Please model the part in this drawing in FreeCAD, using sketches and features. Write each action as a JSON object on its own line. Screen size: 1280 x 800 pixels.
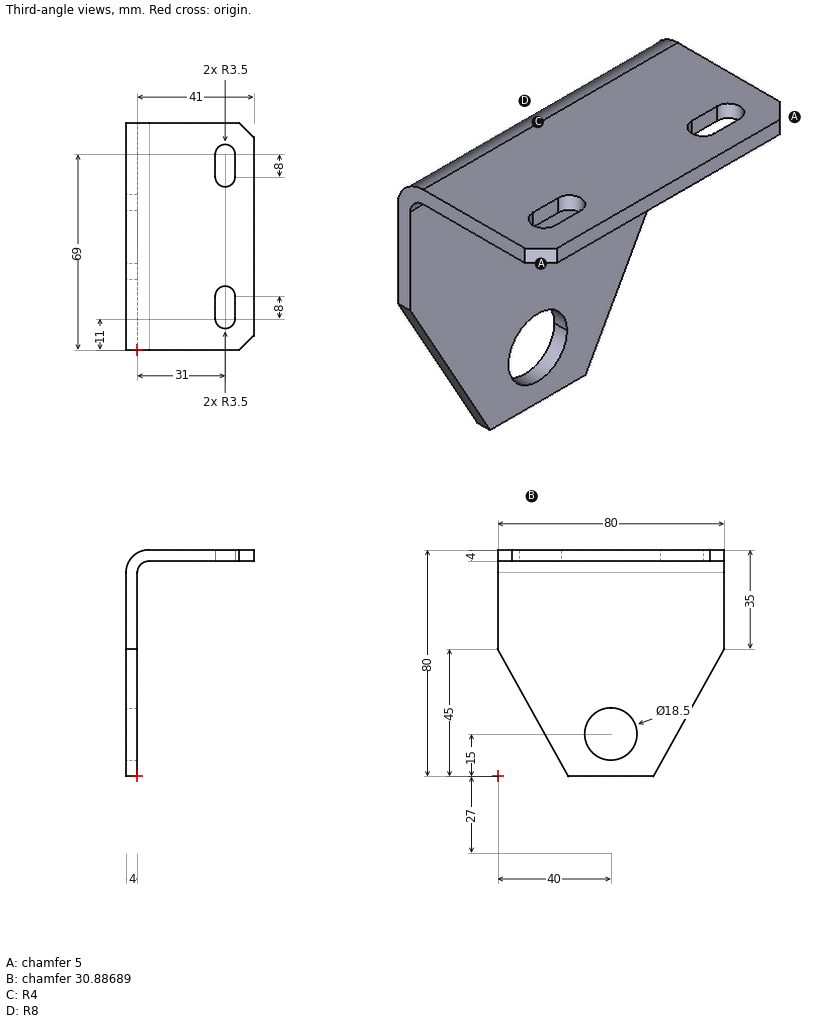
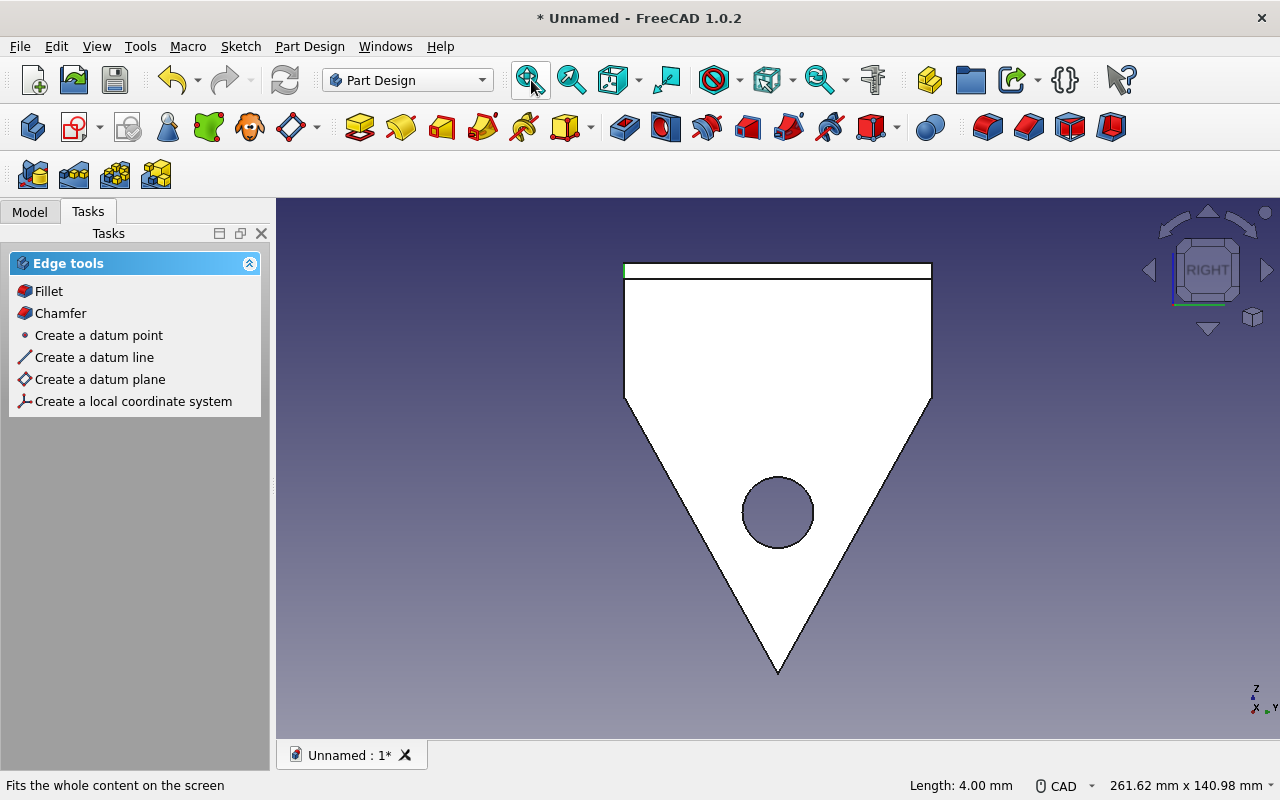
{"action": "left_click", "coordinate": [932, 270], "text": "ctrl"}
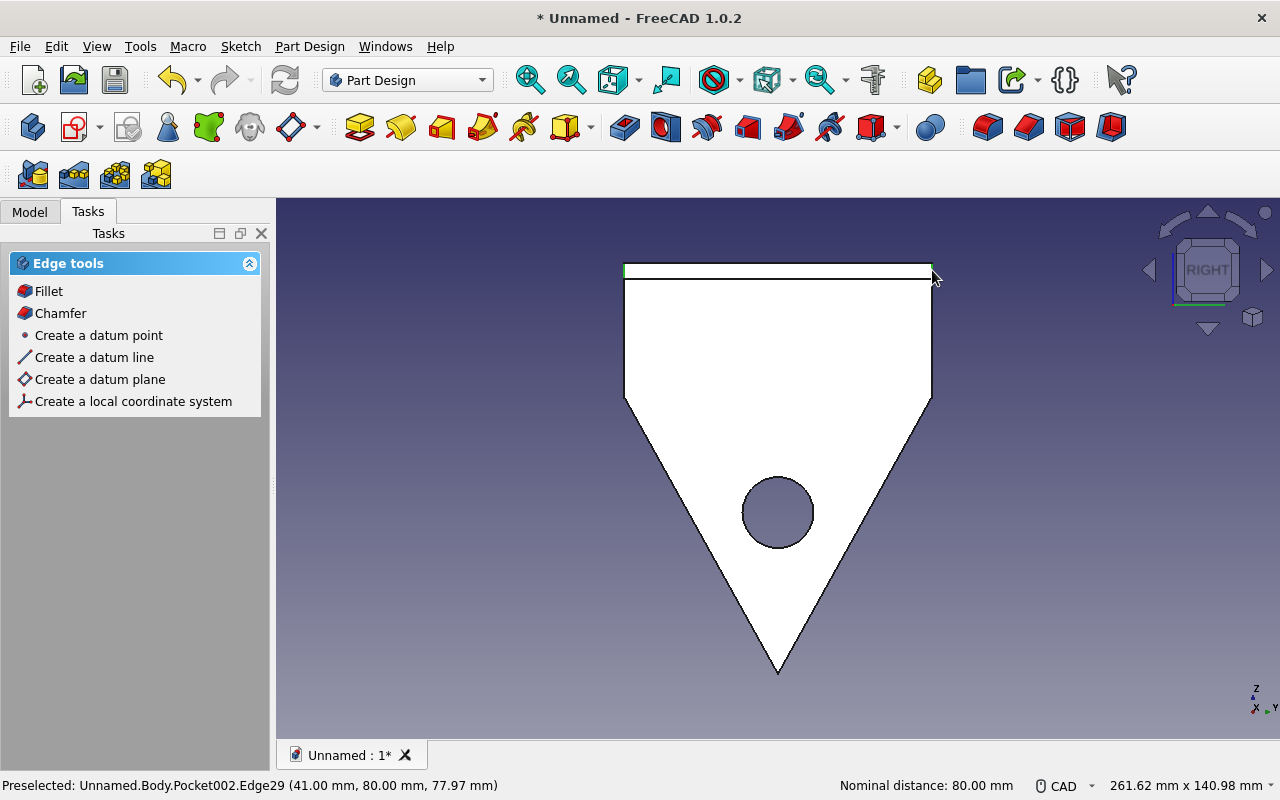
{"action": "left_click", "coordinate": [1029, 128]}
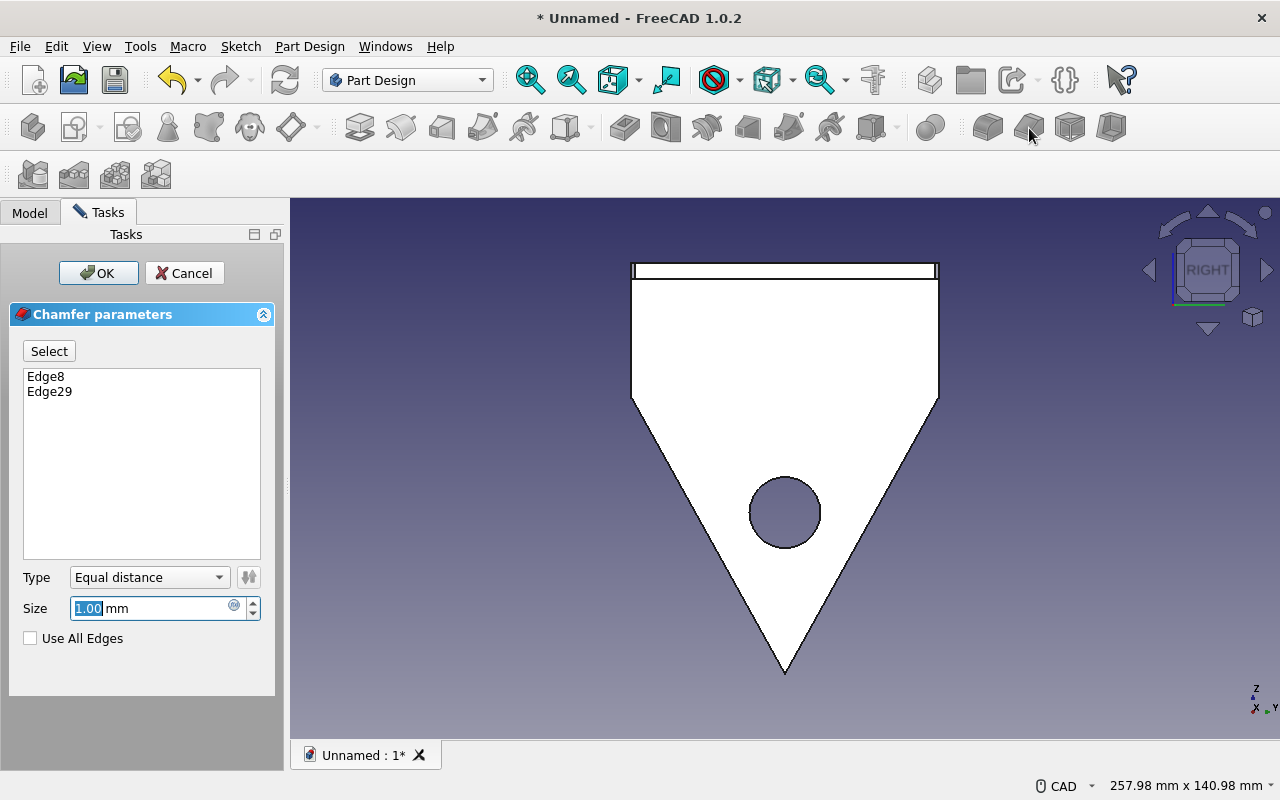
{"action": "type", "text": "5"}
{"action": "key", "text": "Tab"}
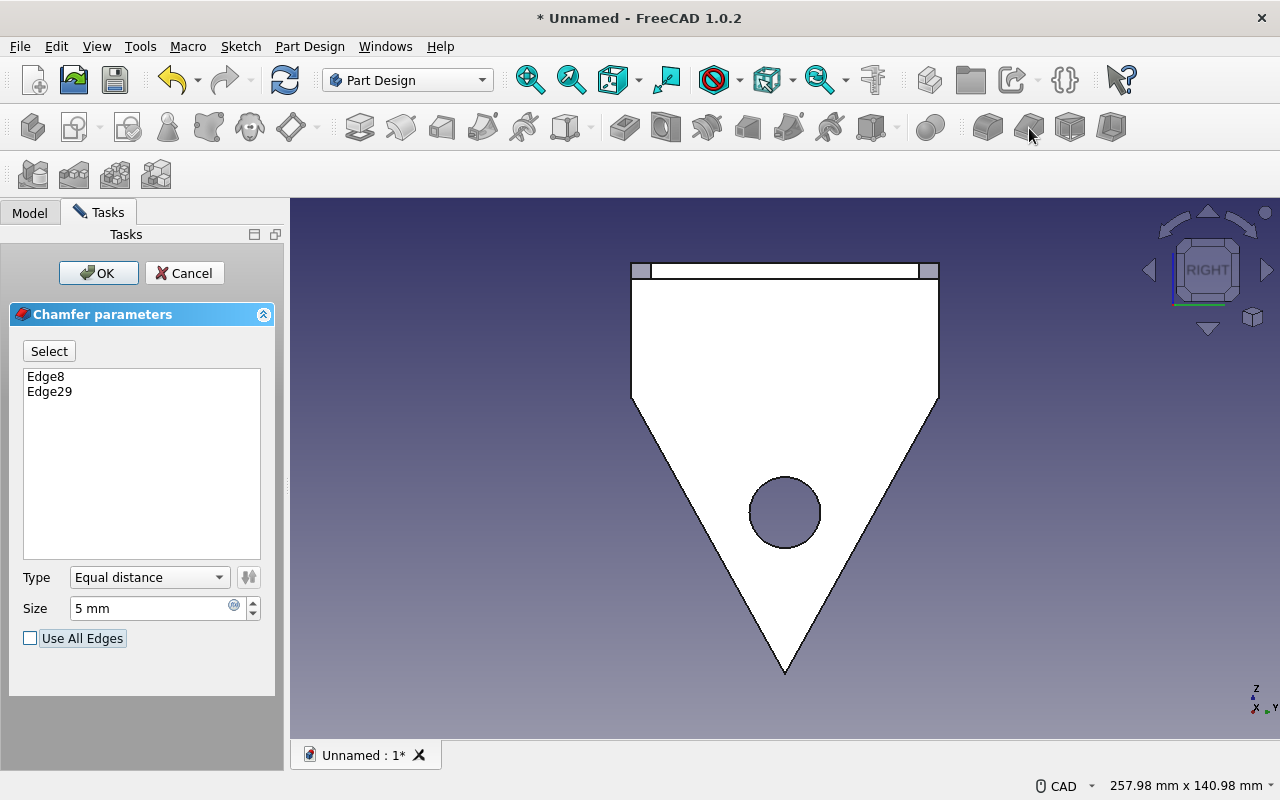
{"action": "left_click", "coordinate": [99, 273]}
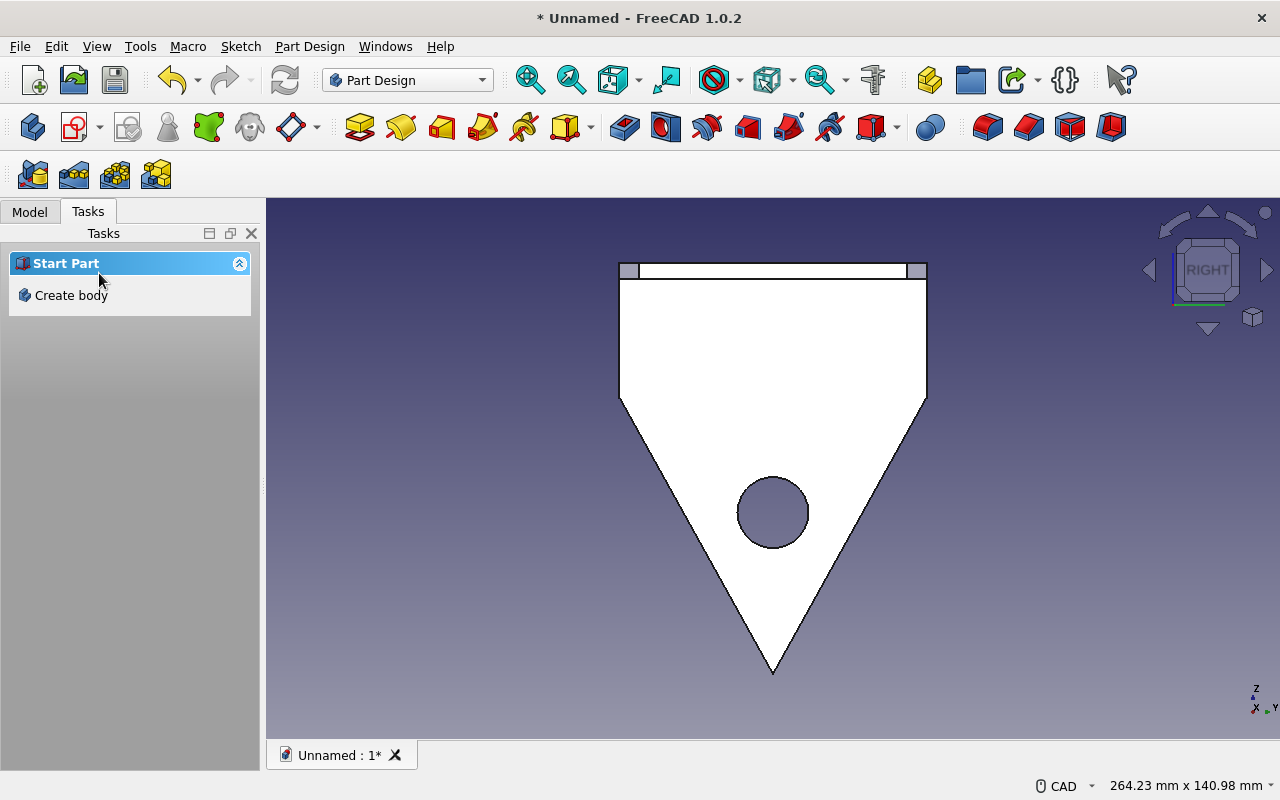
{"action": "scroll", "coordinate": [773, 673], "scroll_direction": "up", "scroll_amount": 5}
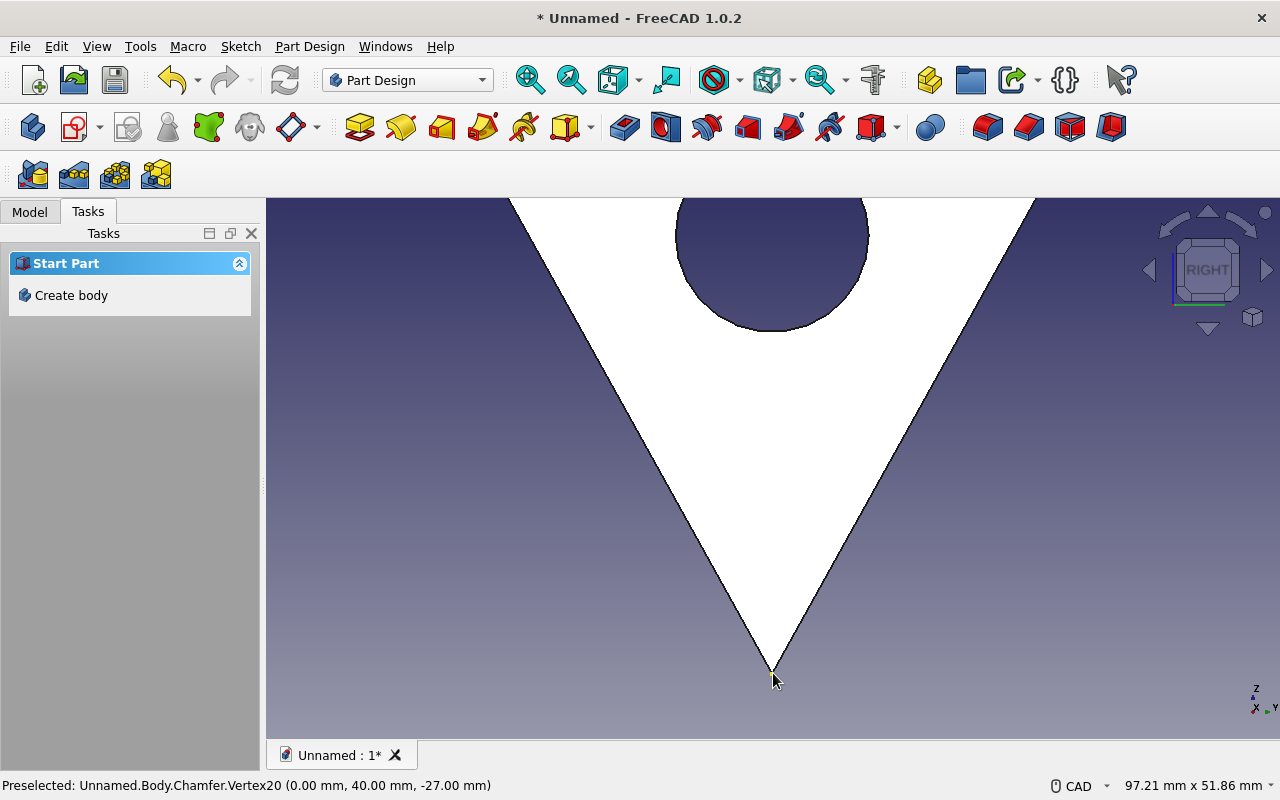
{"action": "key", "text": "v f"}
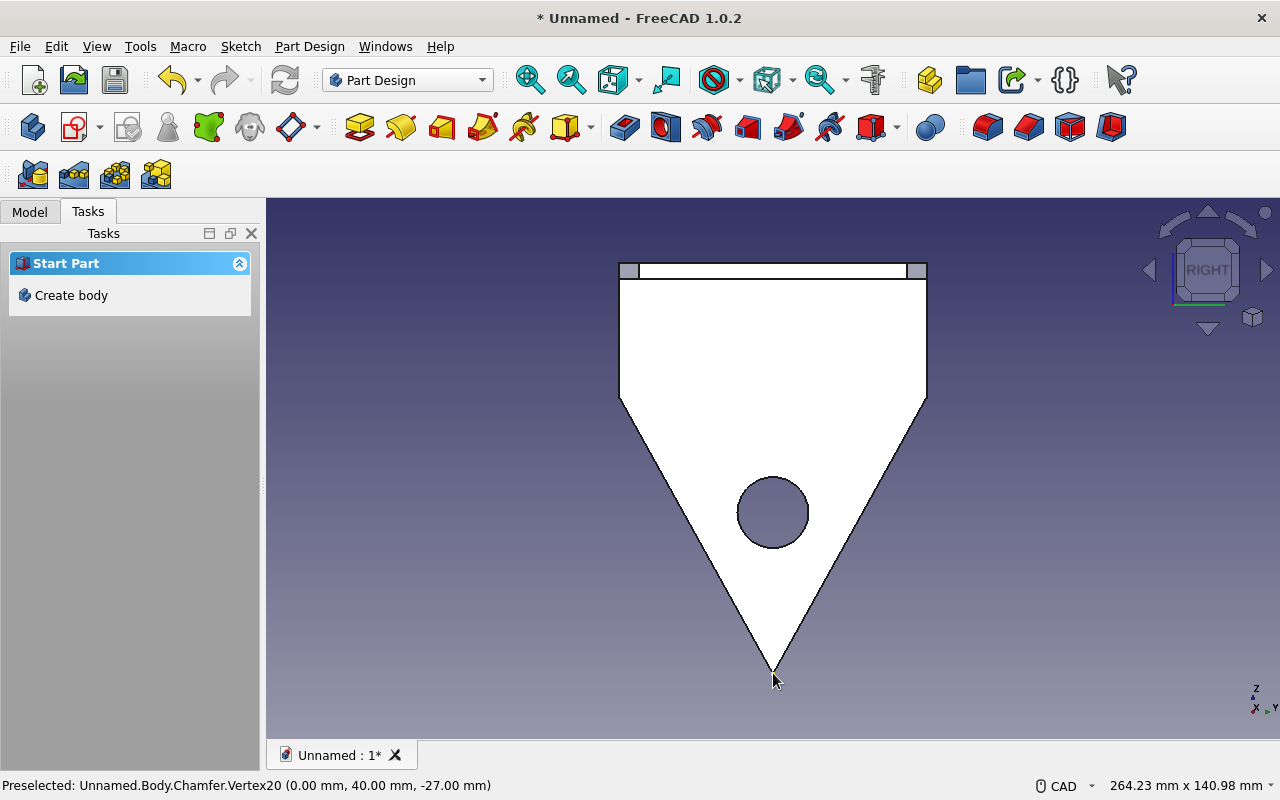
{"action": "key", "text": "0"}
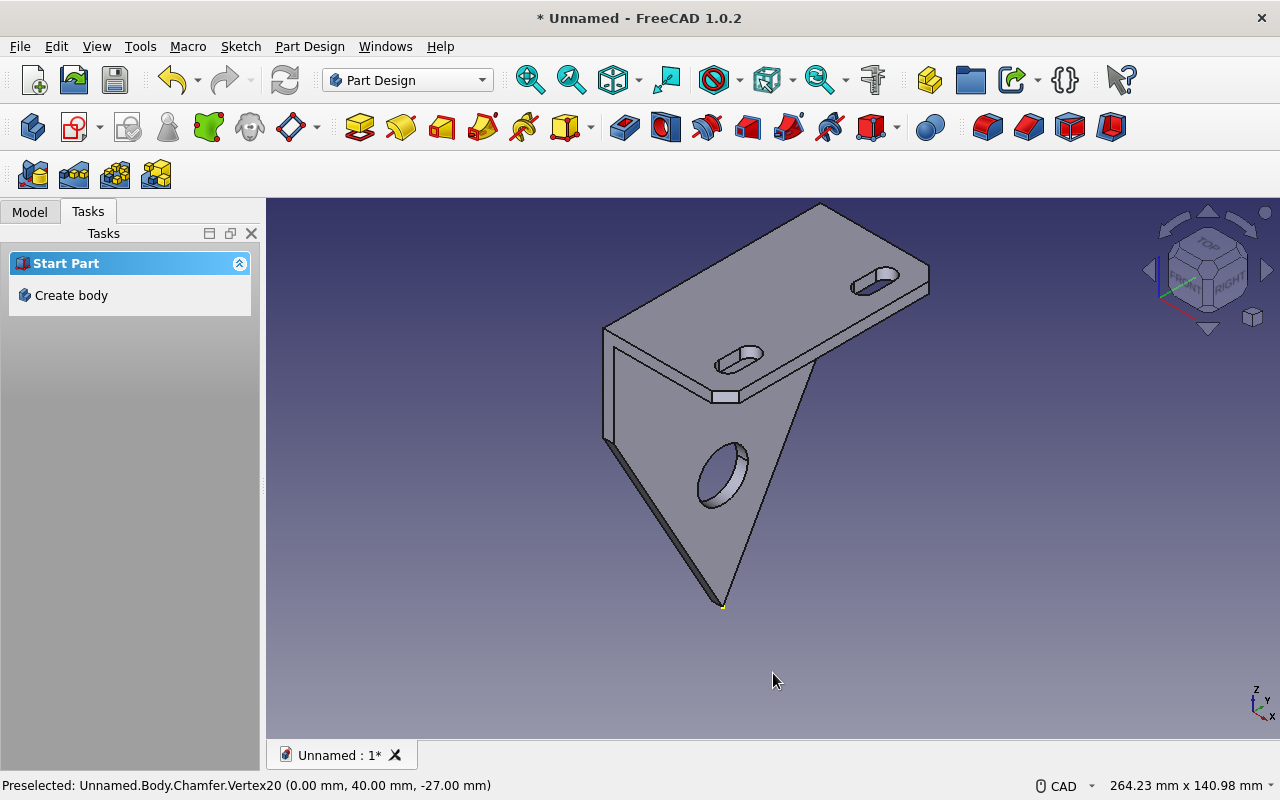
{"action": "scroll", "coordinate": [717, 603], "scroll_direction": "up", "scroll_amount": 5}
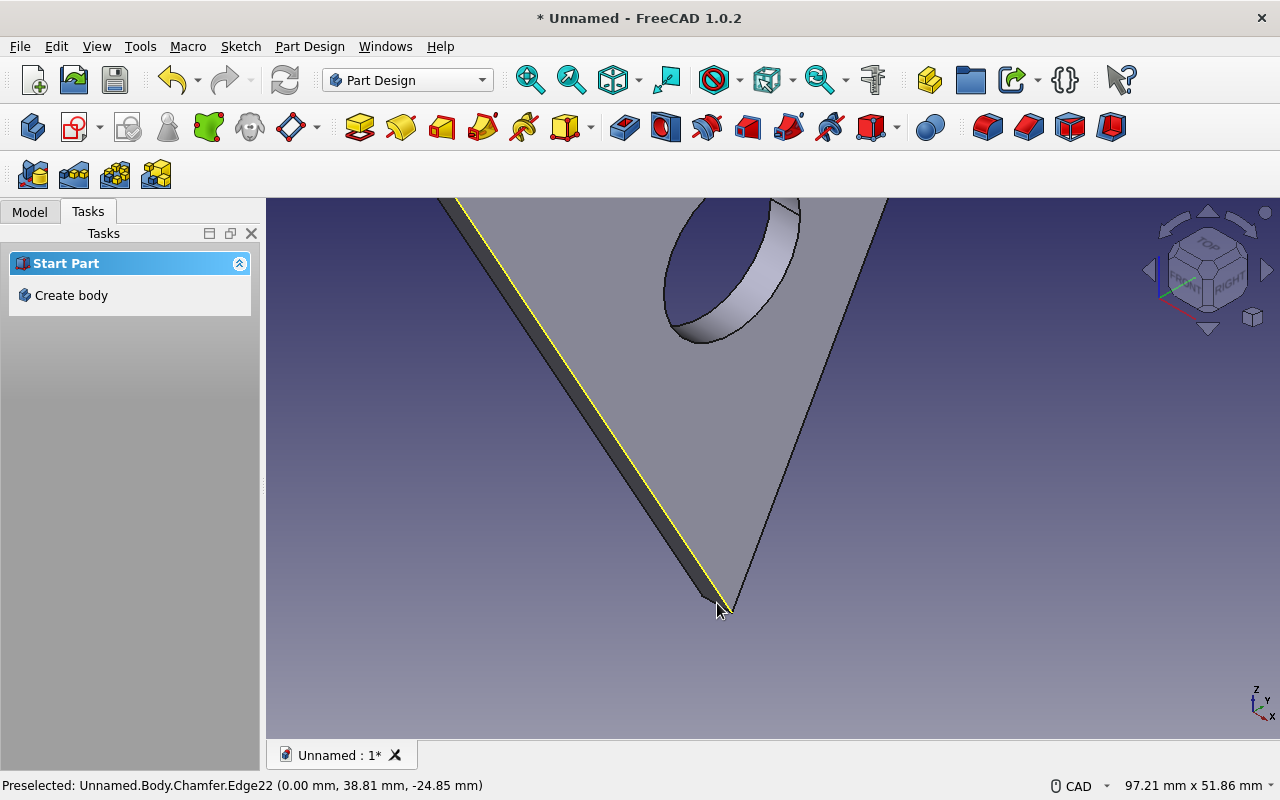
{"action": "key", "text": "v f"}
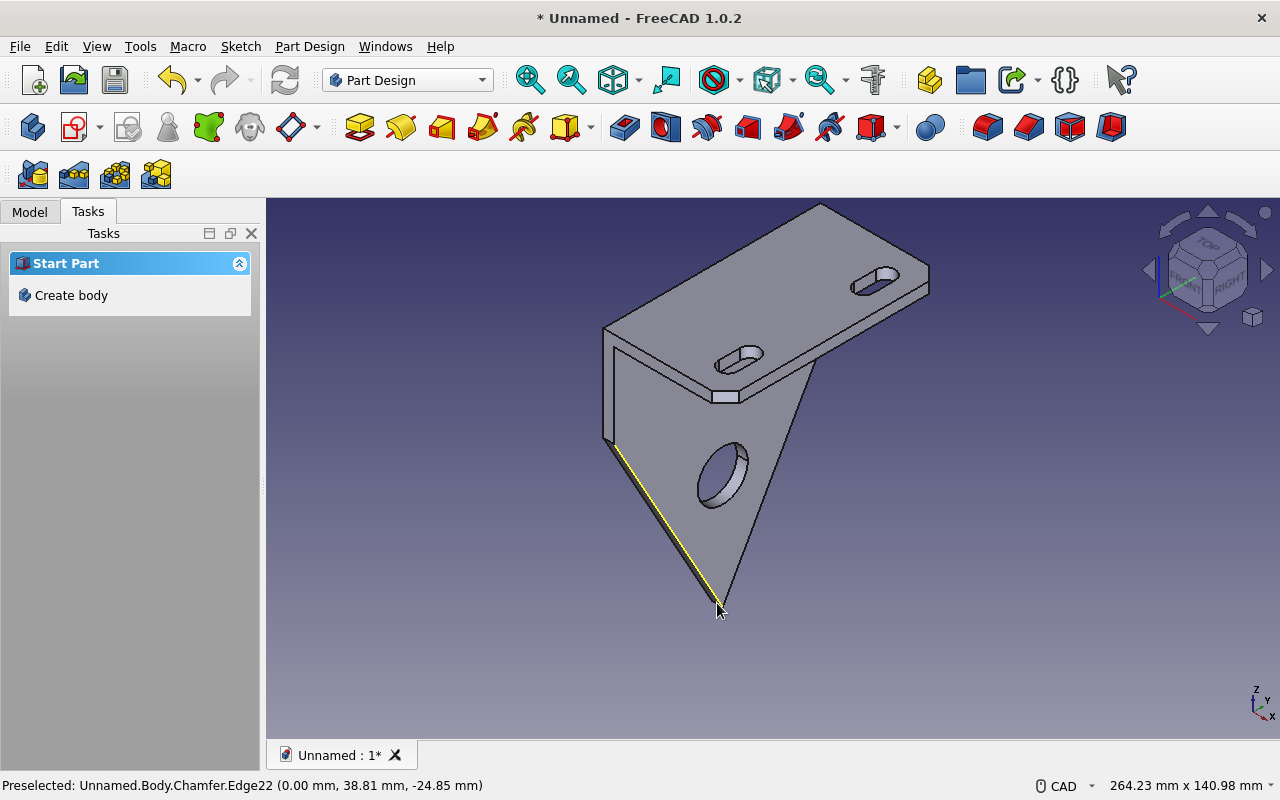
{"action": "key", "text": "2"}